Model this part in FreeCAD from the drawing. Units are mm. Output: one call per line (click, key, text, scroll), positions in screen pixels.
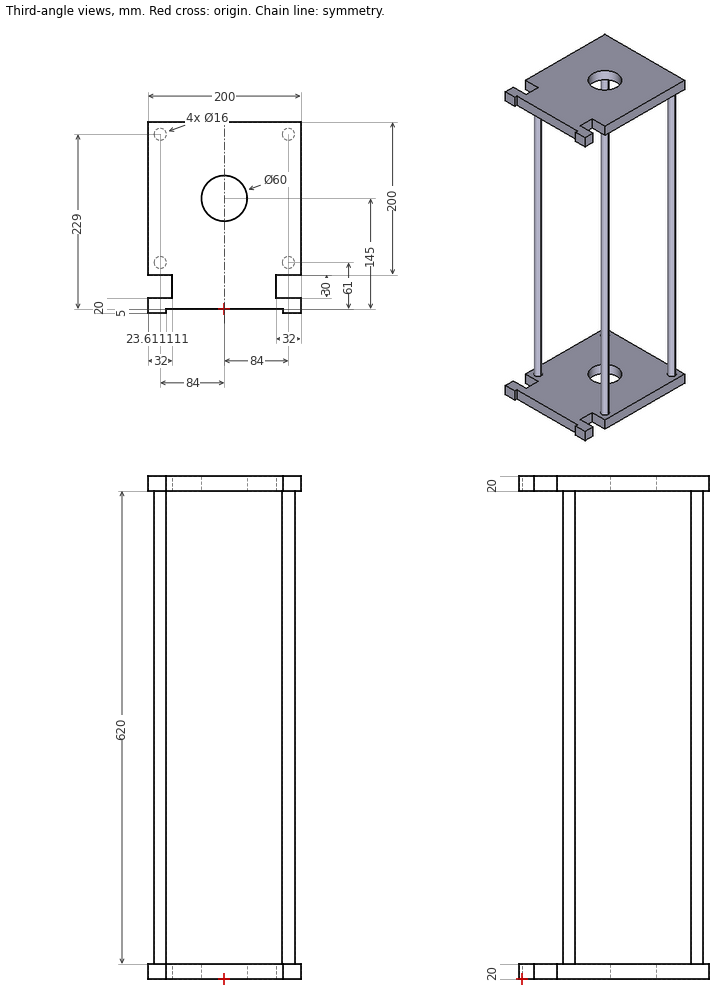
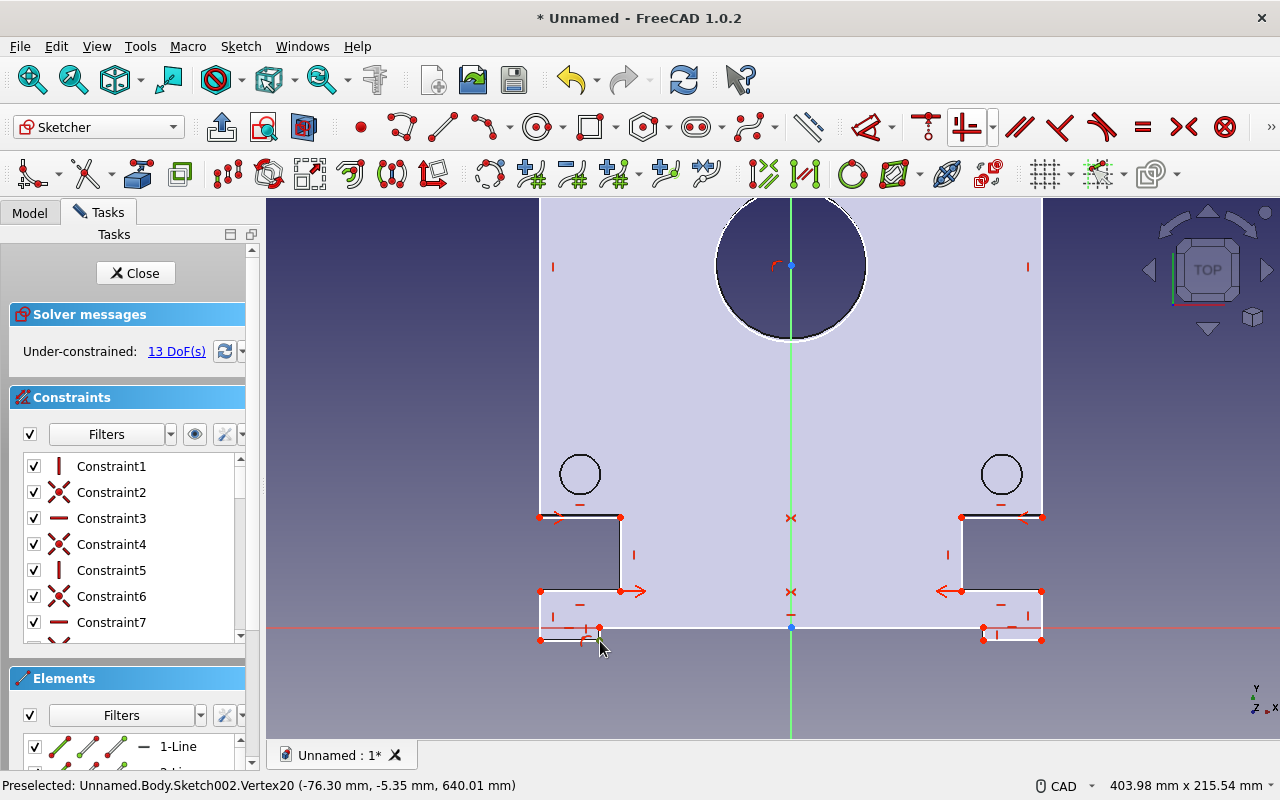
click(984, 640)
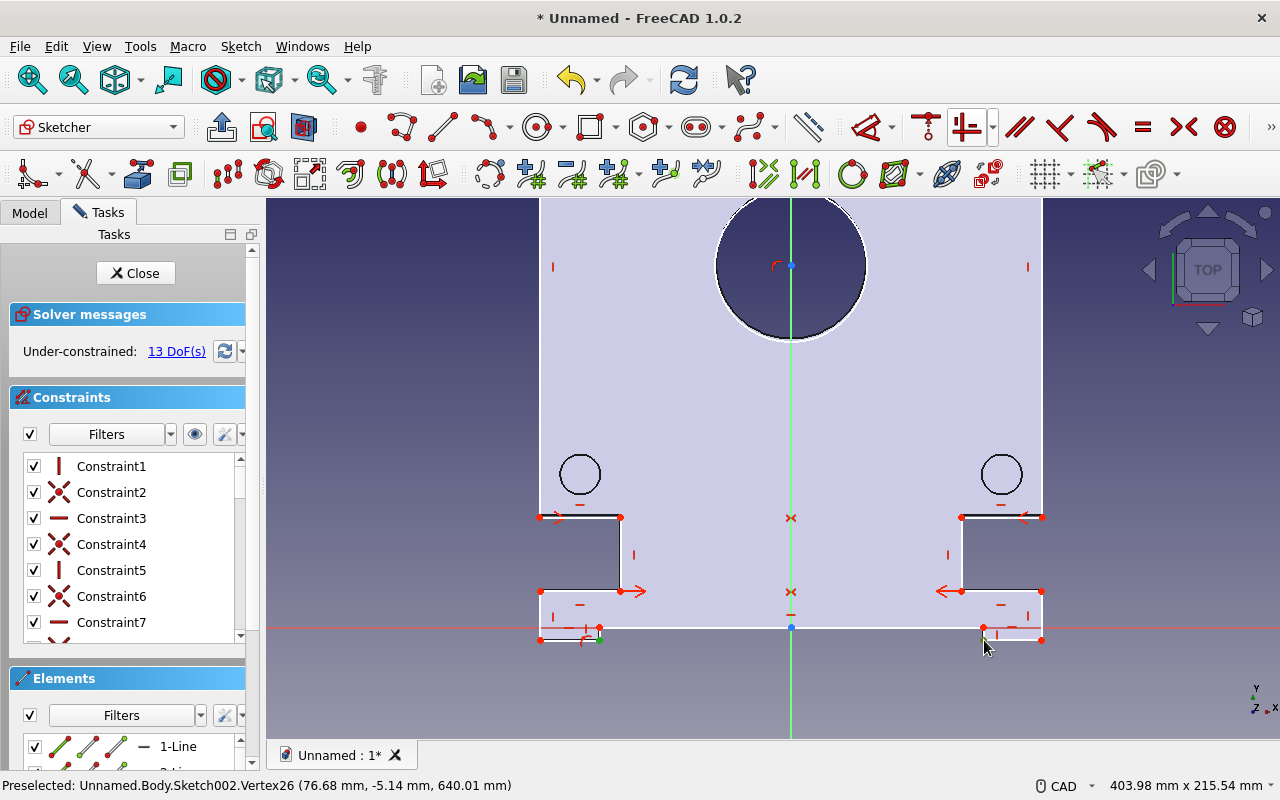
click(791, 676)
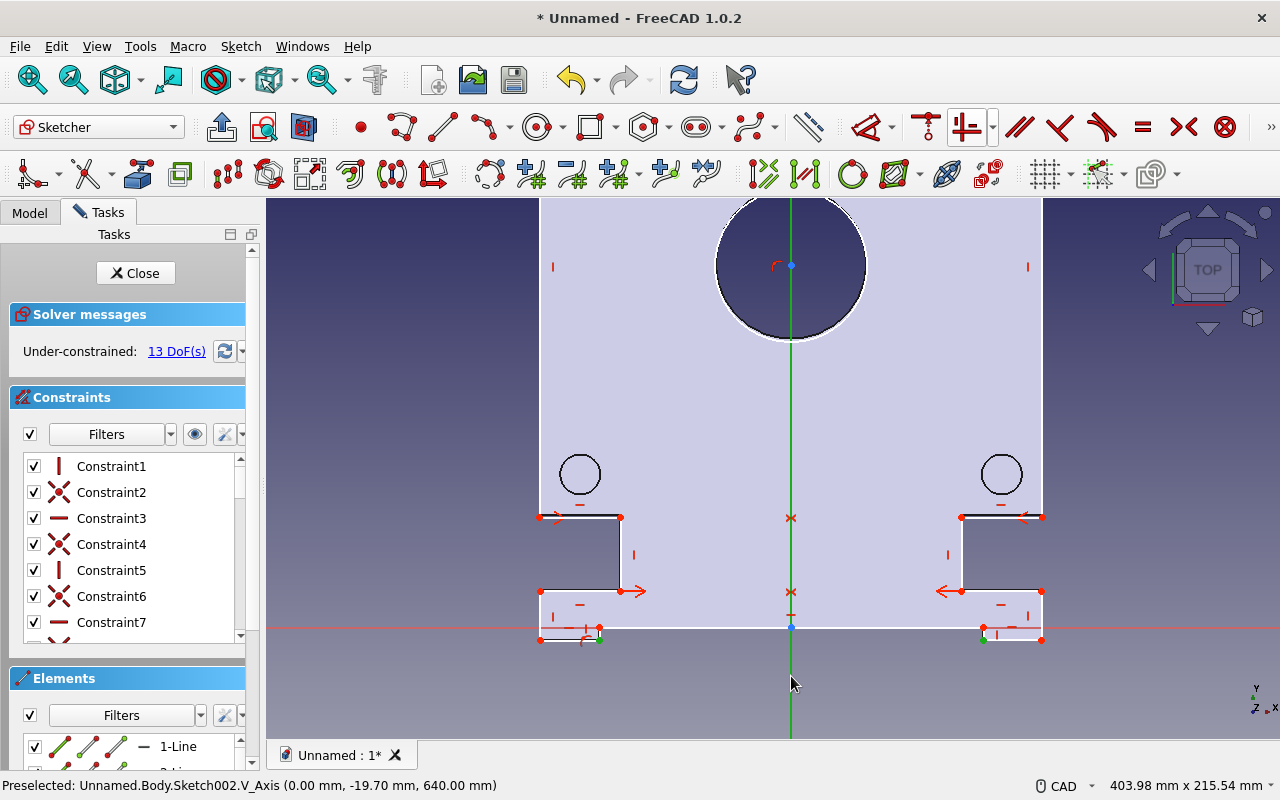
click(1184, 128)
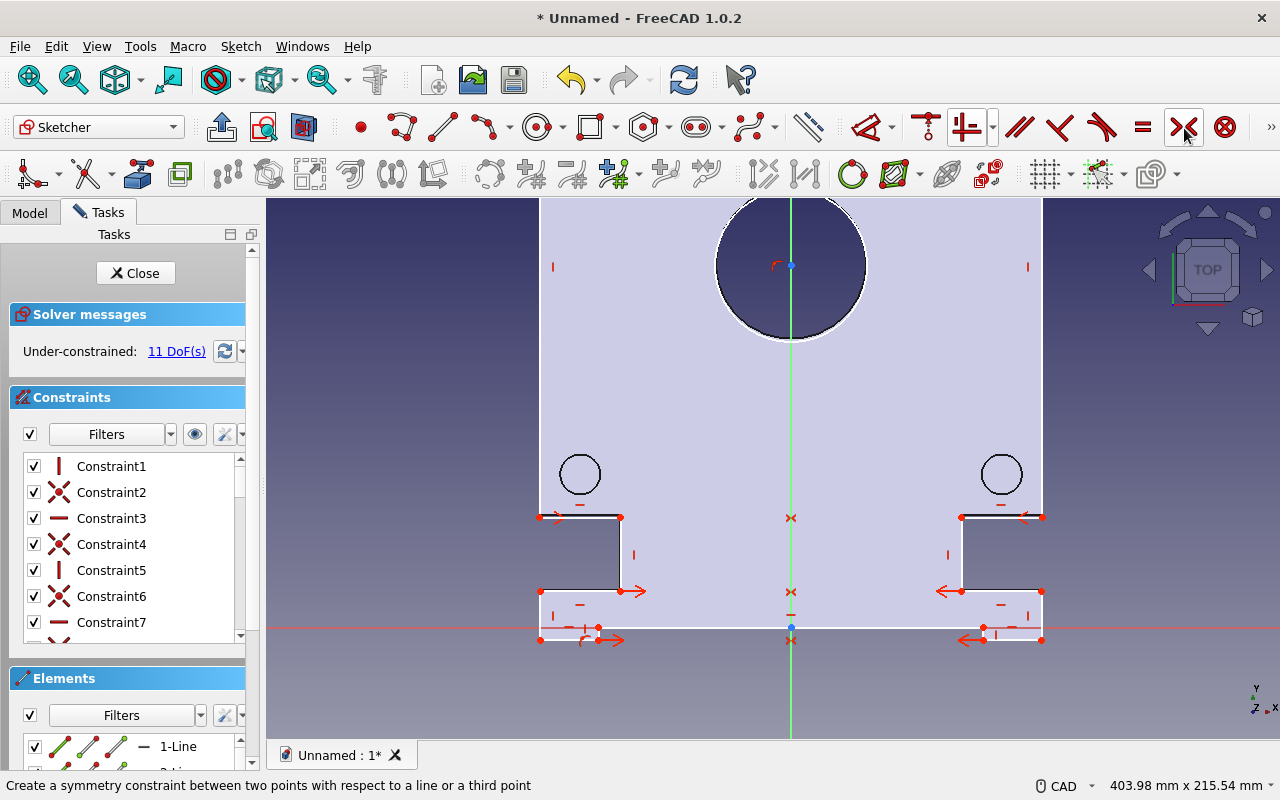
click(866, 128)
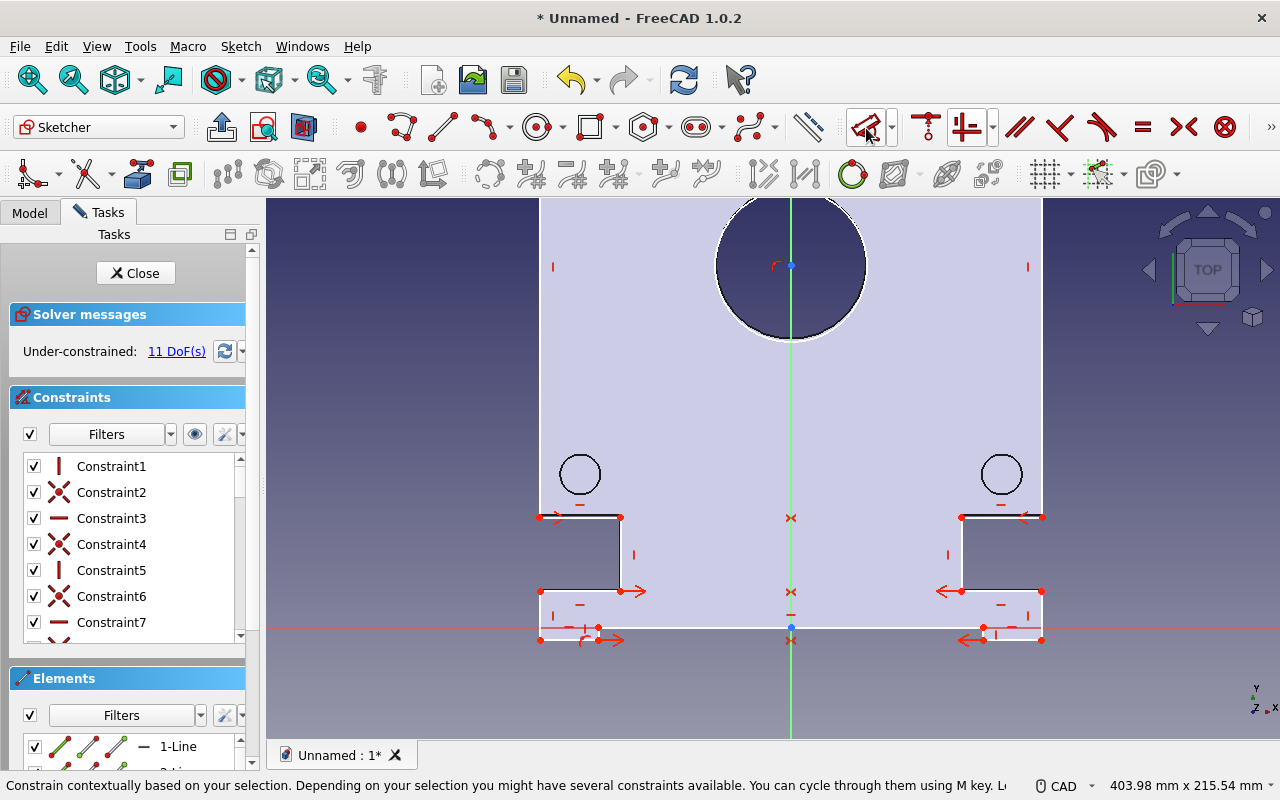
click(737, 320)
click(714, 343)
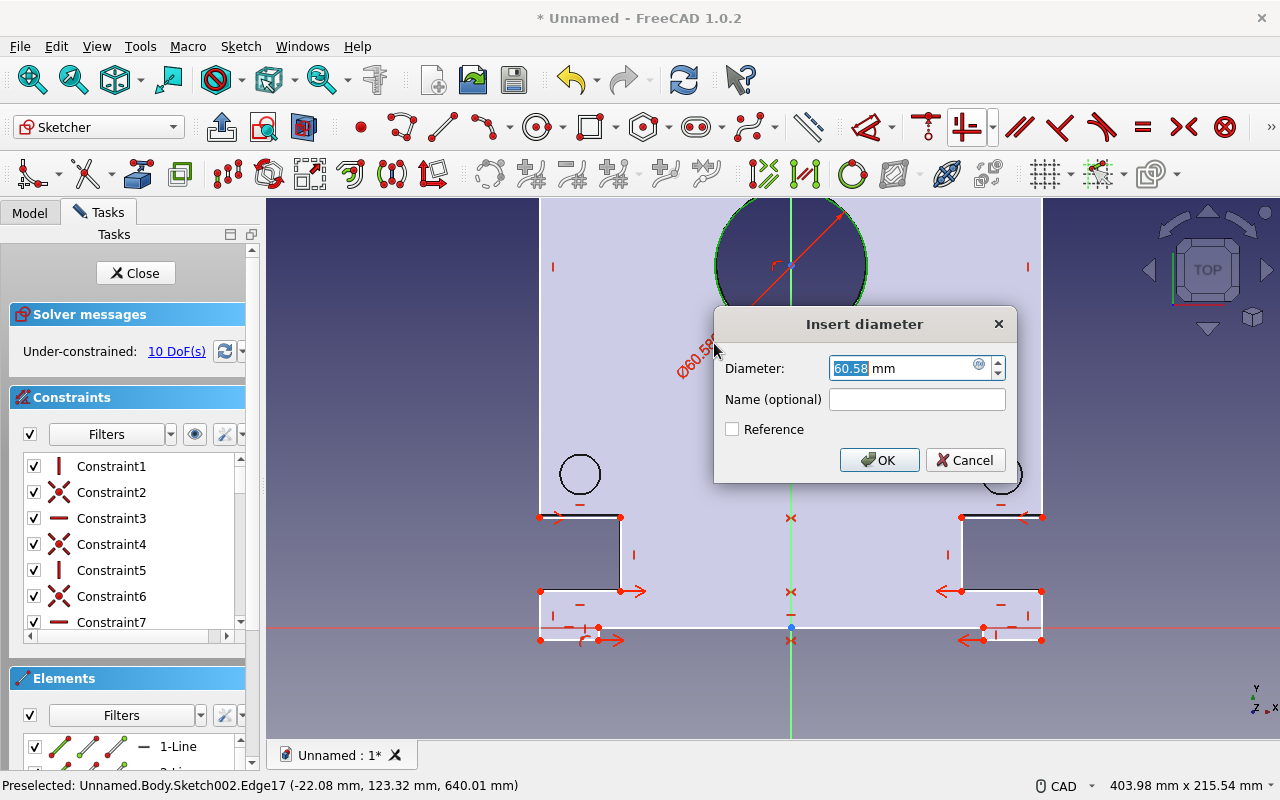
text(60)
key(Return)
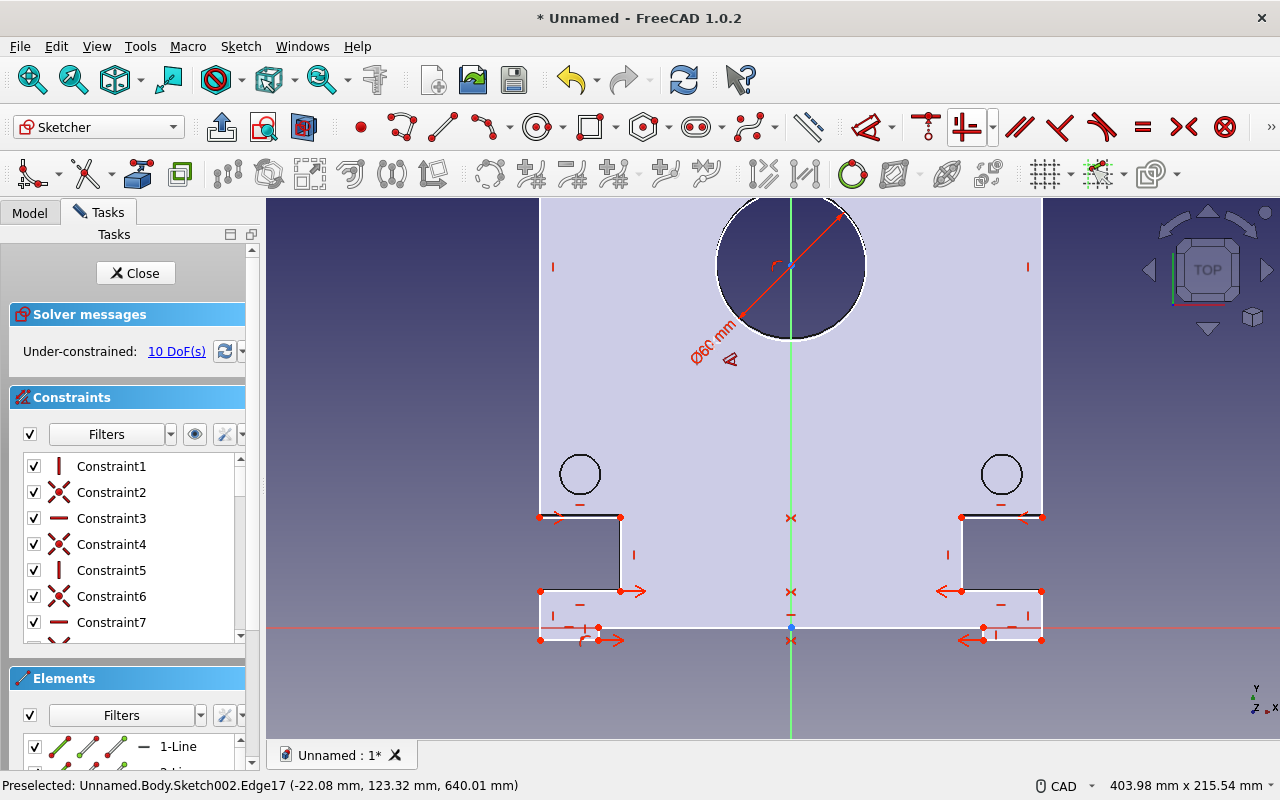
scroll(599, 634, up, 6)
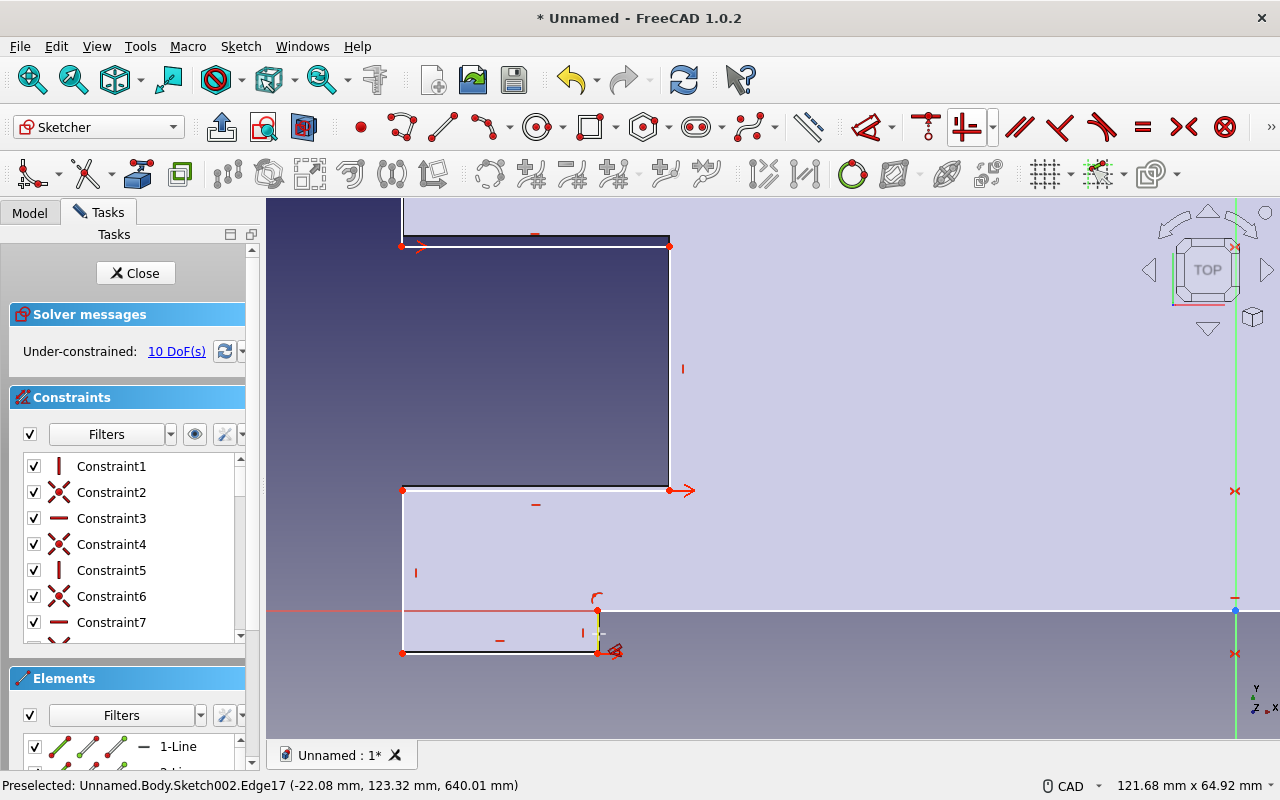
click(598, 632)
click(564, 632)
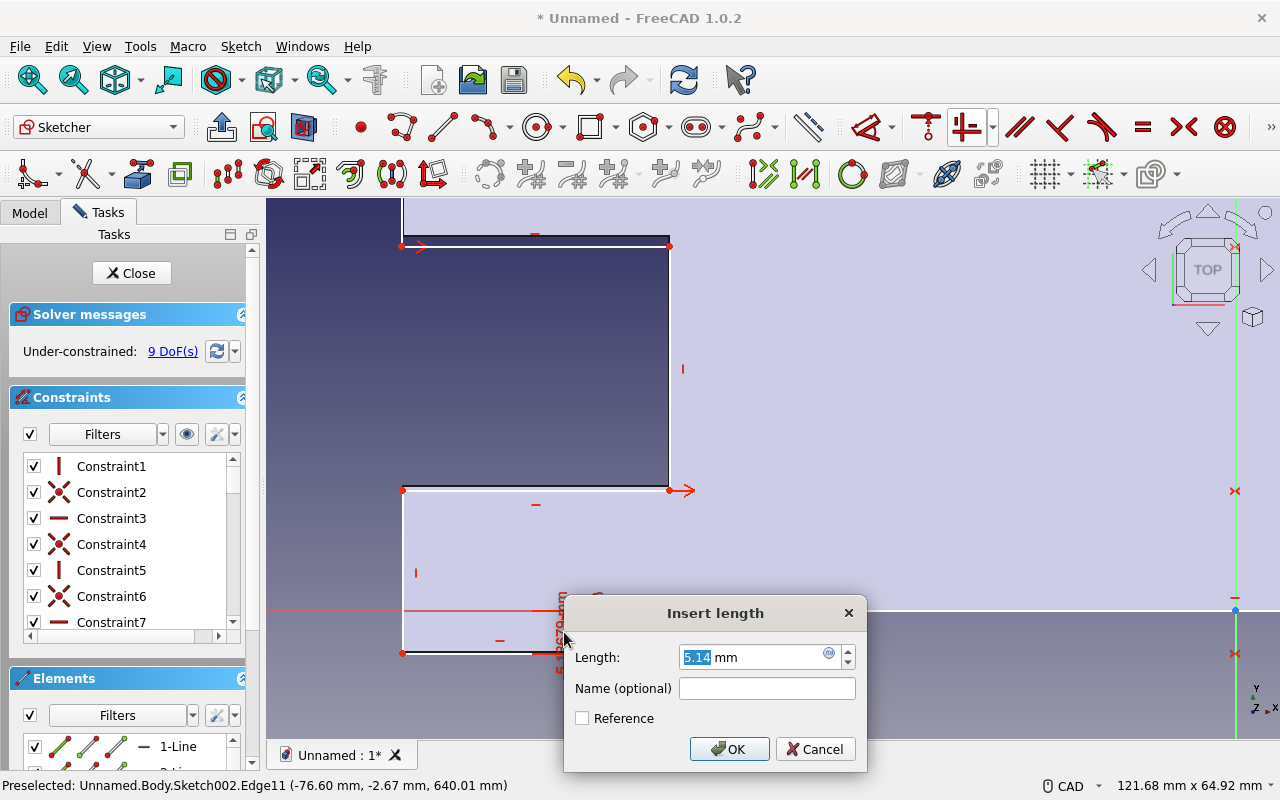
text(5)
key(Return)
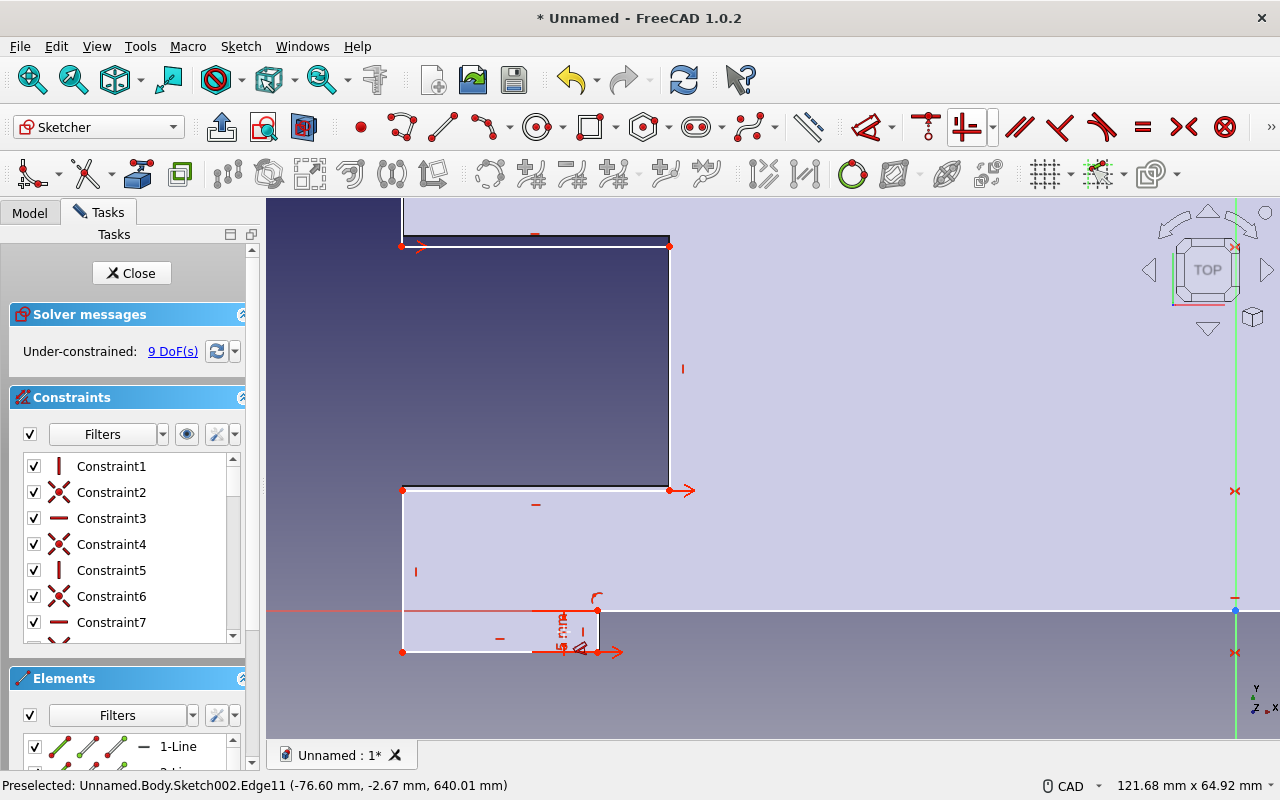
scroll(599, 638, down, 9)